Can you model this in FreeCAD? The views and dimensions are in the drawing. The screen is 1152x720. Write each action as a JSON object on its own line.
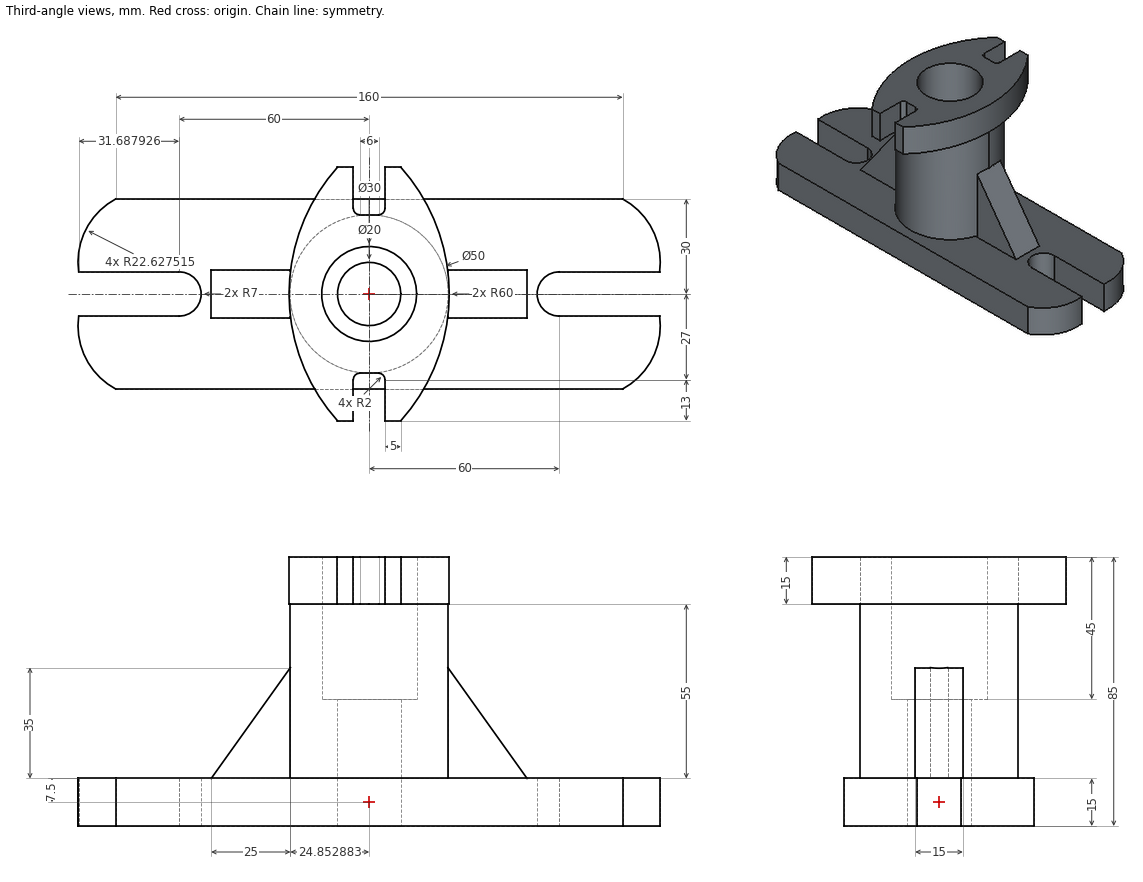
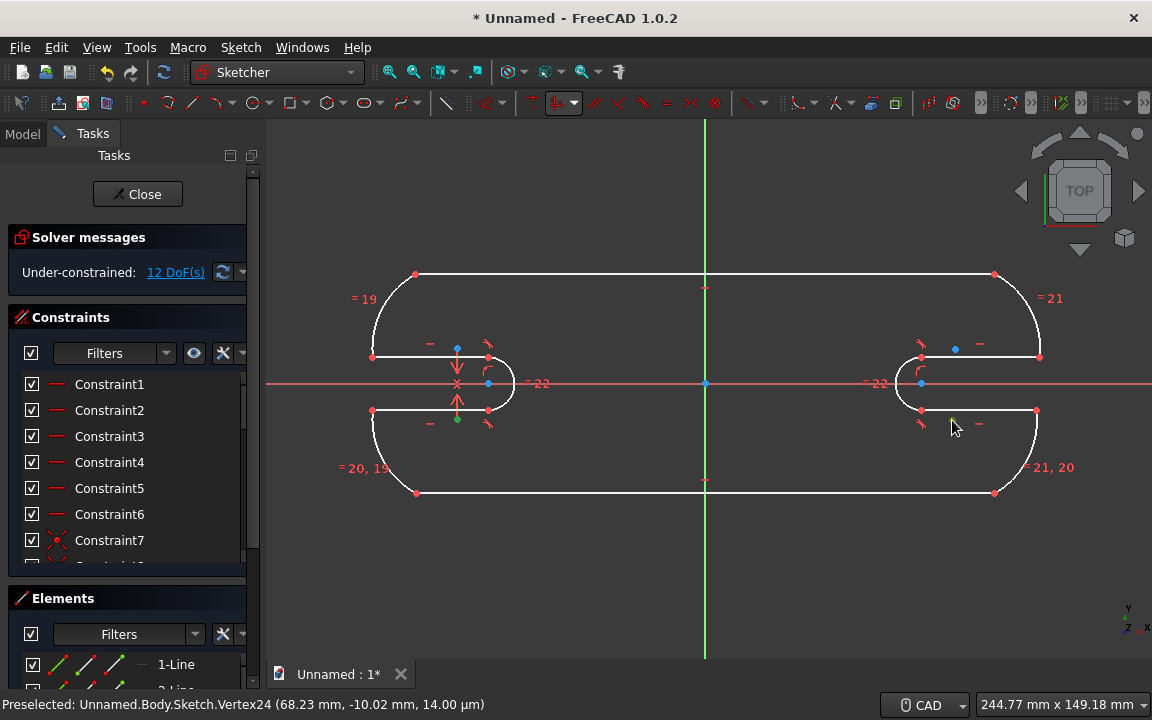
{"action": "left_click", "coordinate": [705, 596]}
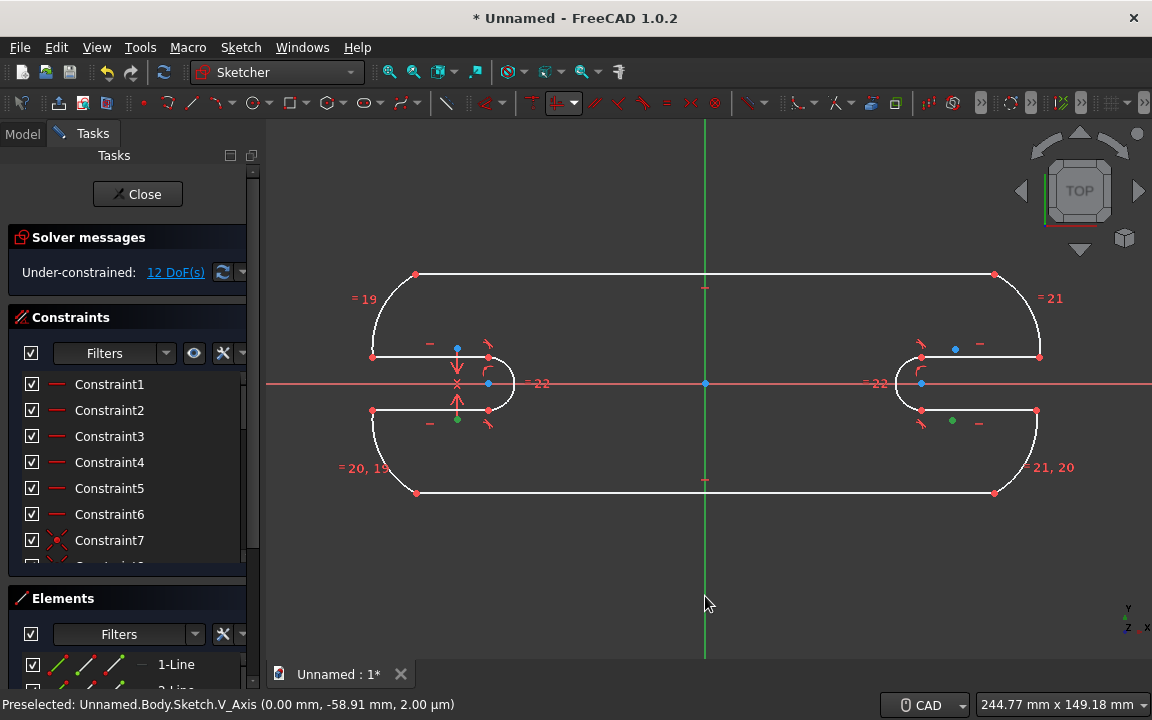
{"action": "key", "text": "s"}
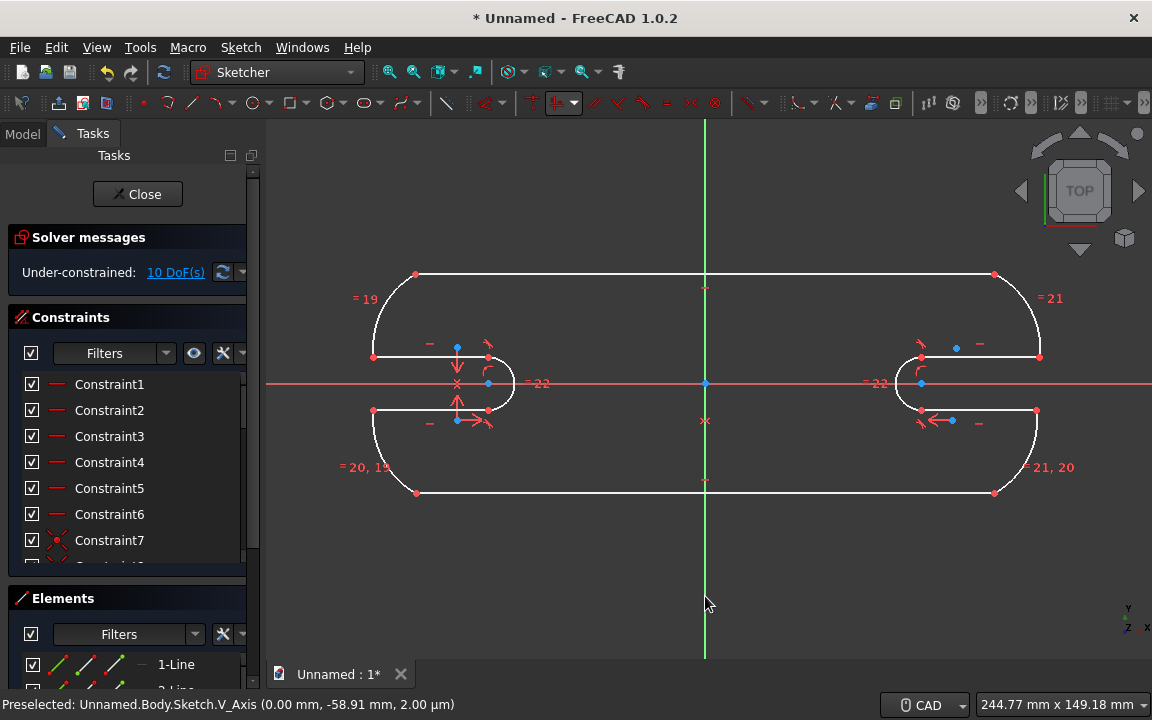
{"action": "left_click", "coordinate": [457, 347]}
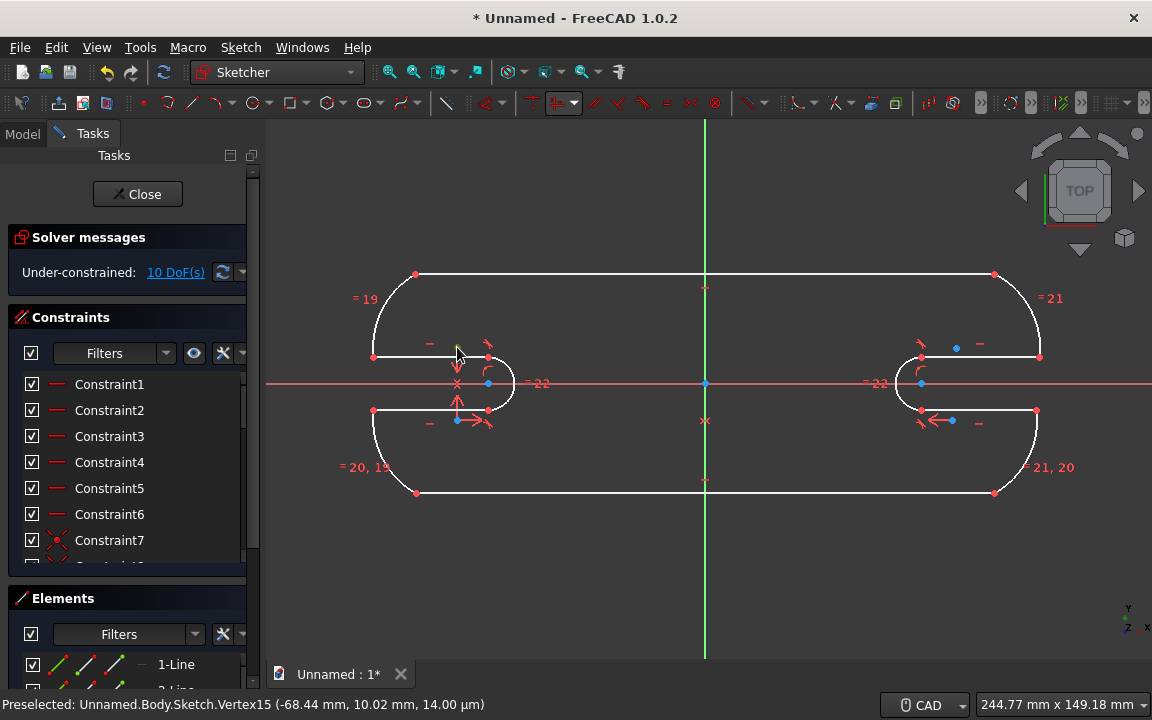
{"action": "left_click", "coordinate": [956, 349]}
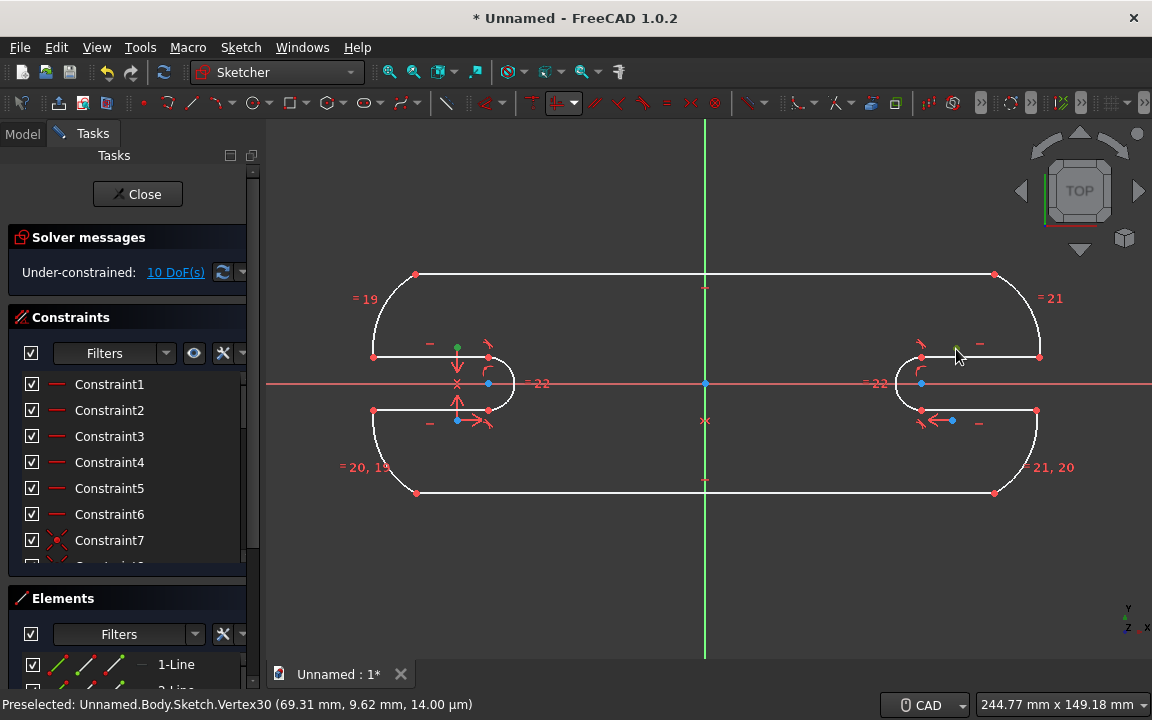
{"action": "left_click", "coordinate": [705, 596]}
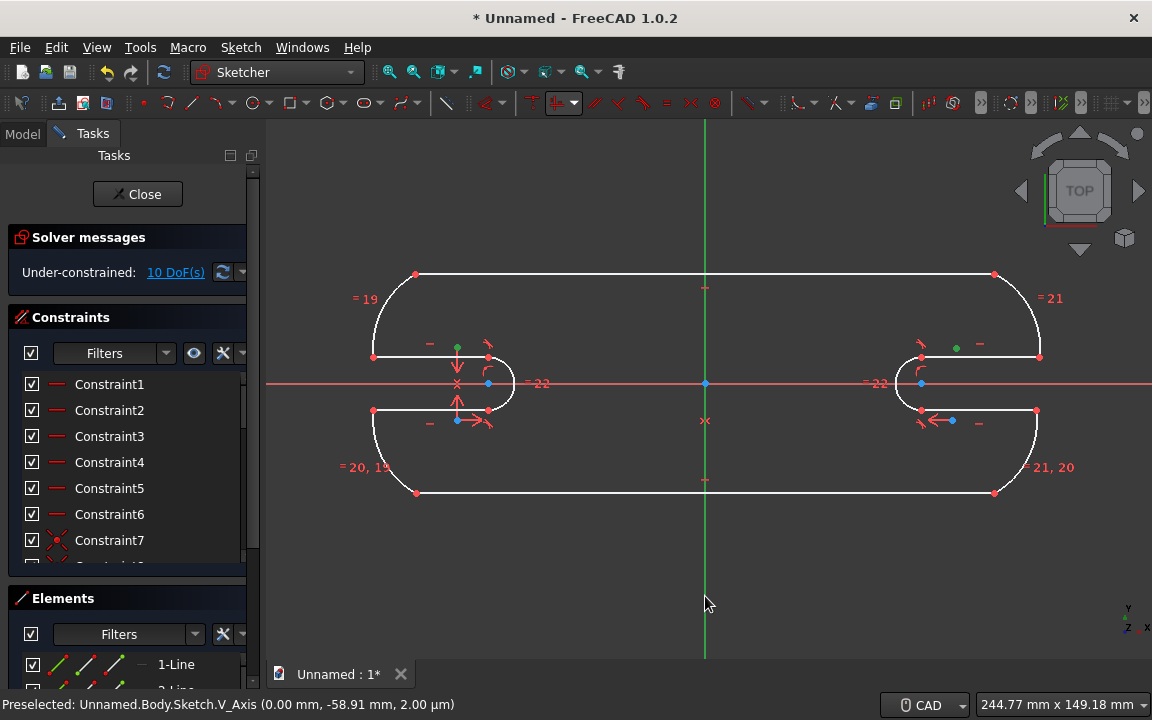
{"action": "key", "text": "s"}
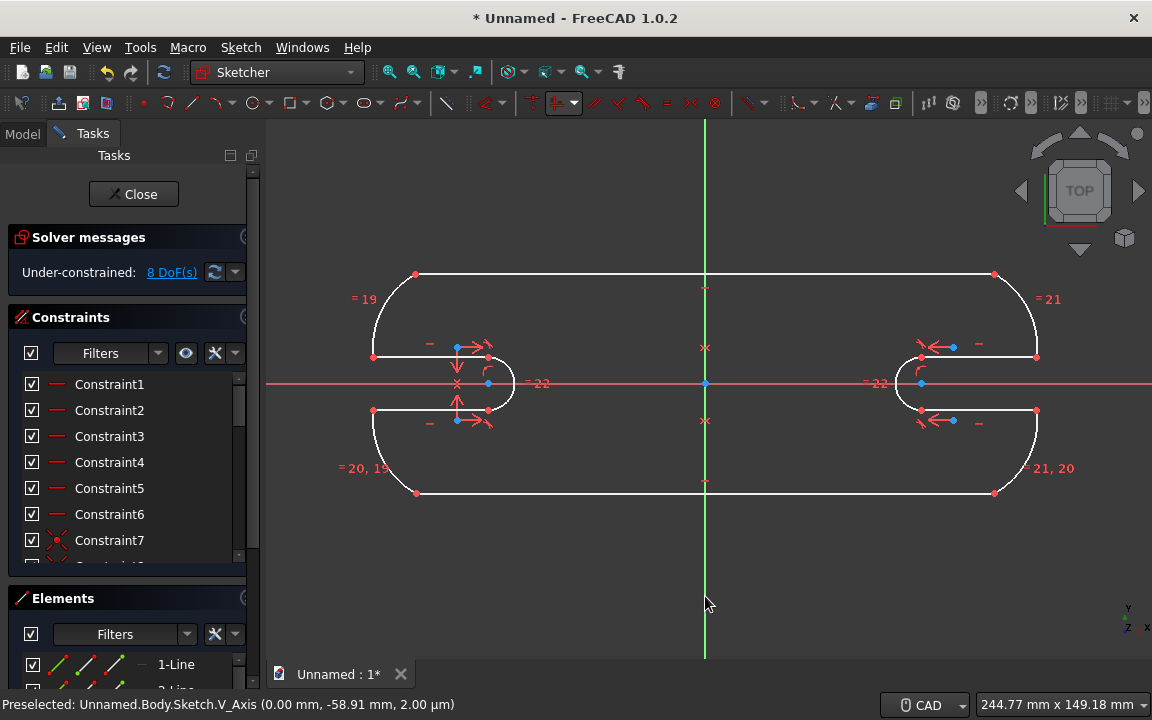
{"action": "left_click", "coordinate": [486, 104]}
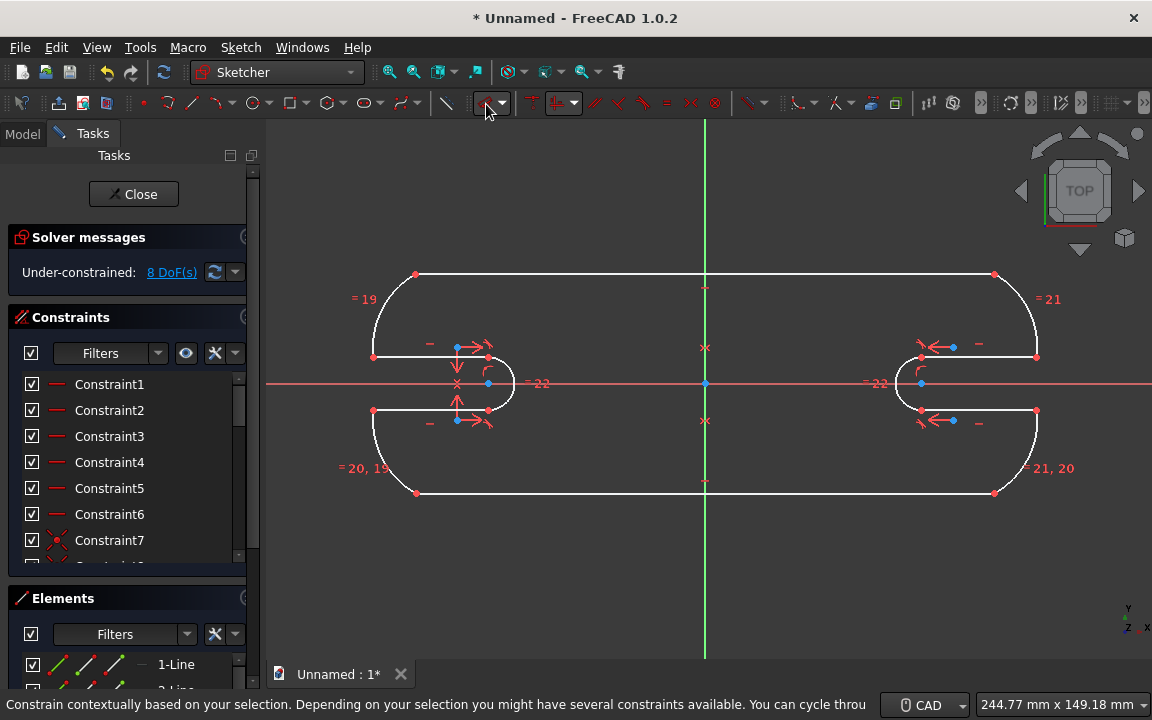
{"action": "left_click", "coordinate": [393, 293]}
{"action": "left_click", "coordinate": [369, 272]}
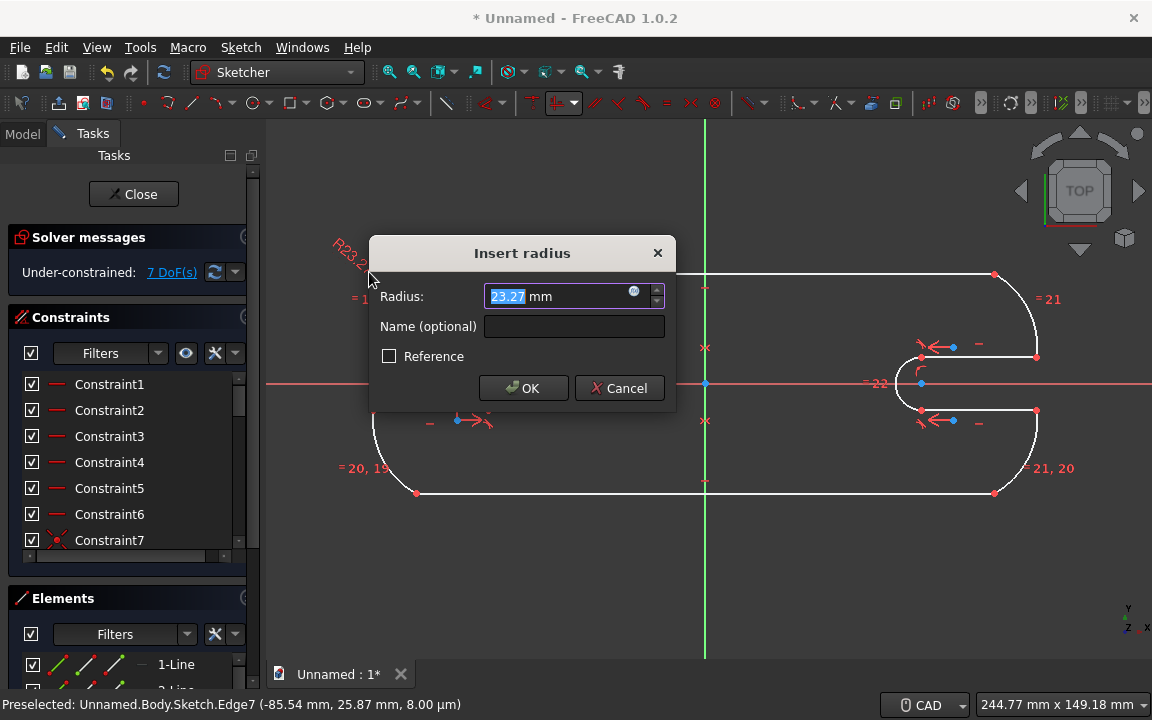
{"action": "type", "text": "22.627515"}
{"action": "key", "text": "Return"}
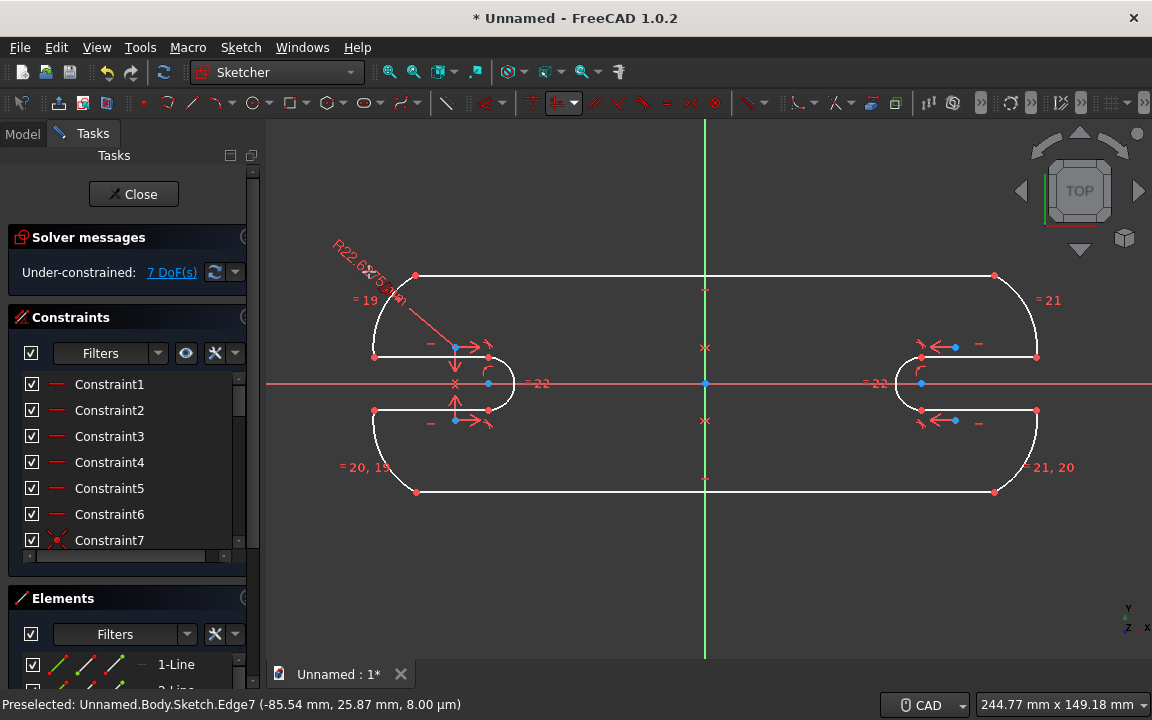
{"action": "scroll", "coordinate": [509, 399], "scroll_direction": "up", "scroll_amount": 3}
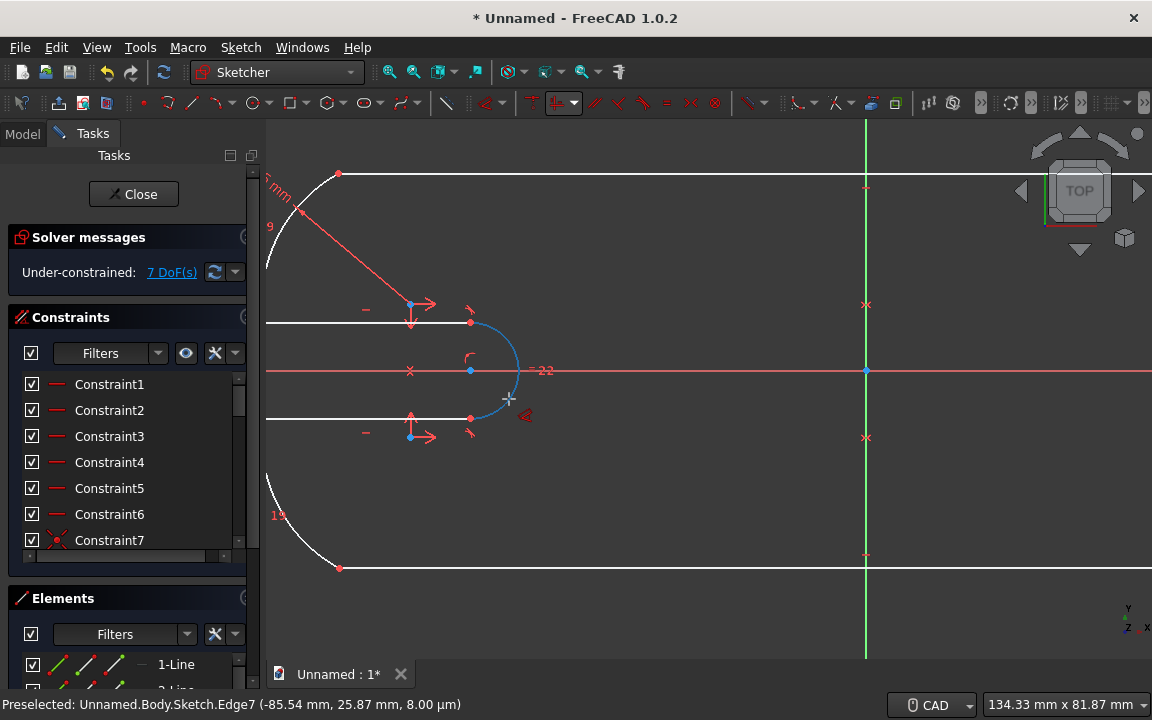
{"action": "left_click", "coordinate": [510, 399]}
{"action": "left_click", "coordinate": [536, 418]}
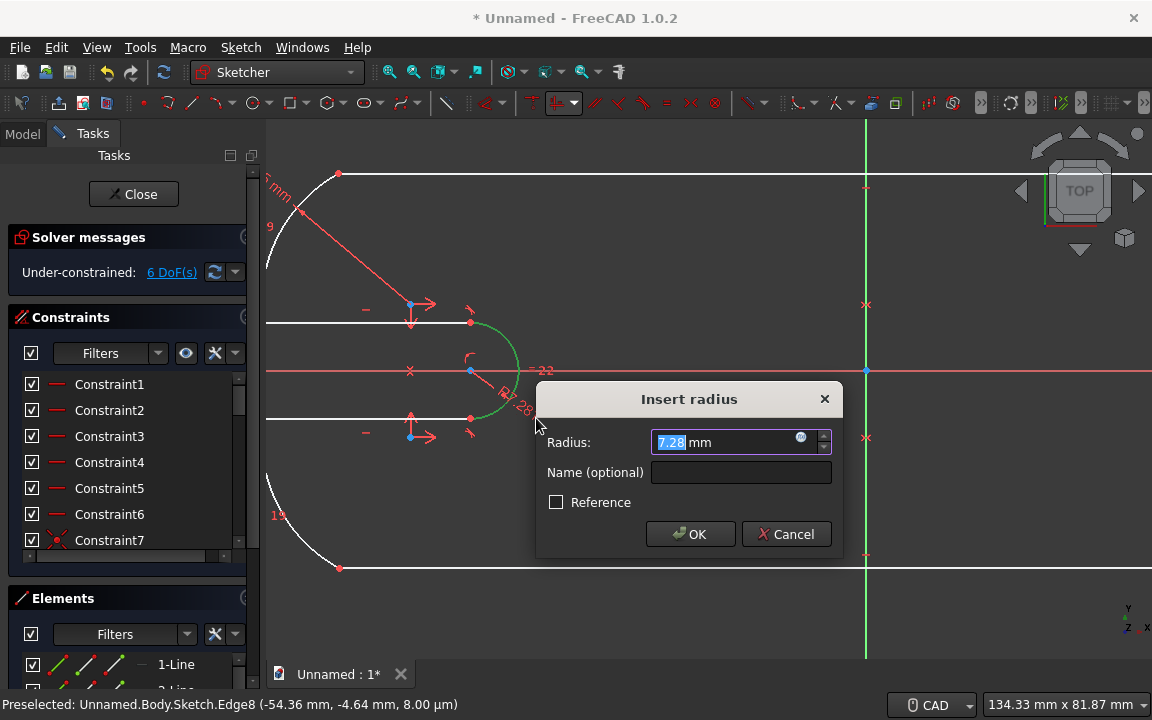
{"action": "type", "text": "7"}
{"action": "key", "text": "Return"}